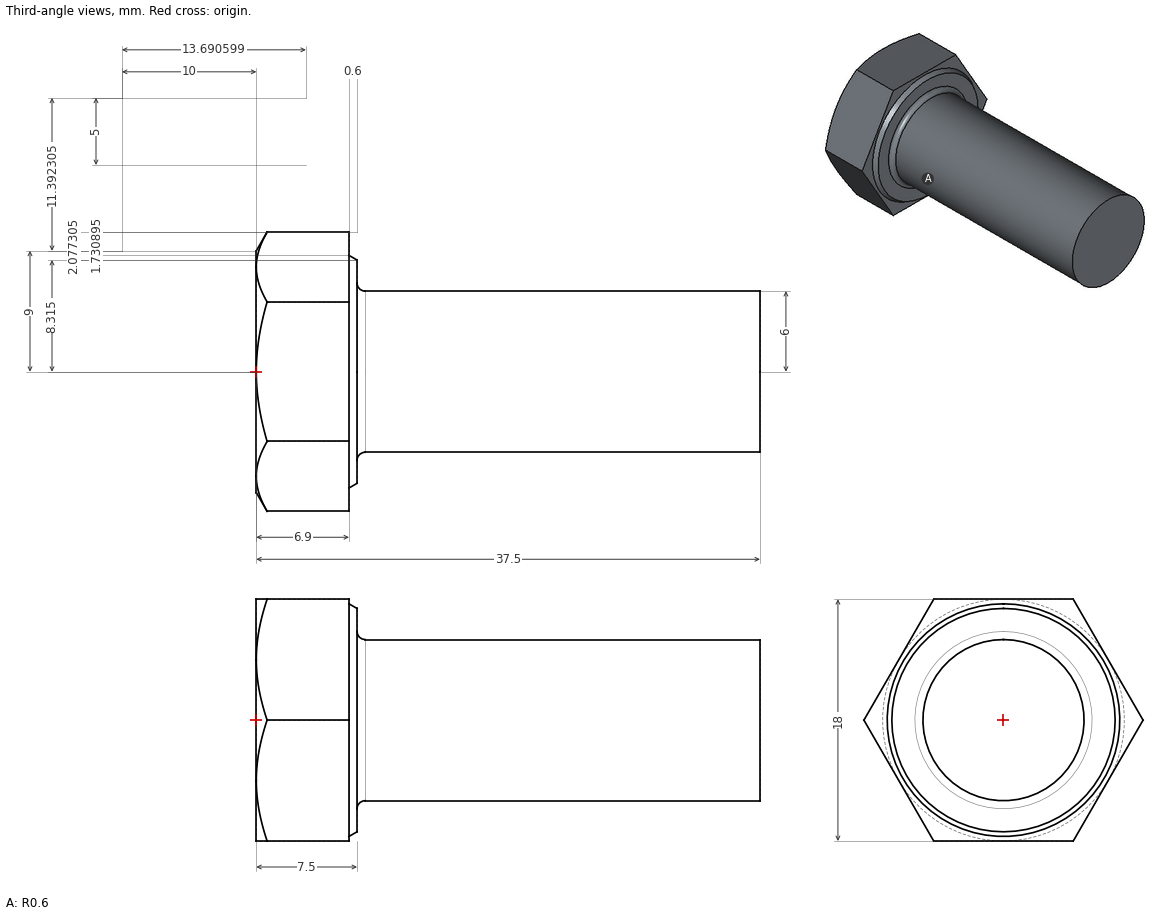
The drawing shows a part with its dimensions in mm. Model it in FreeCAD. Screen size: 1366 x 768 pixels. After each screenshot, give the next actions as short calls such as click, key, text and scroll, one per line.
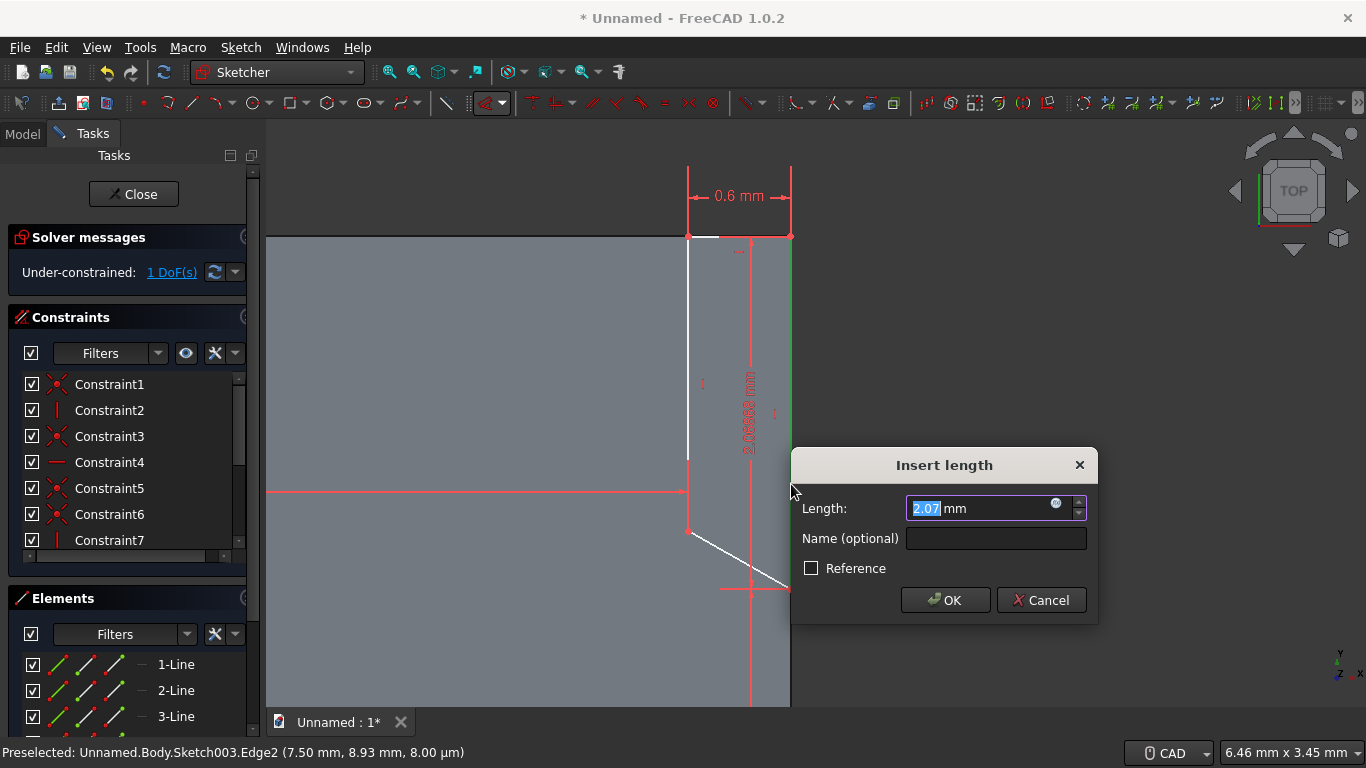
text(2.077305)
key(Return)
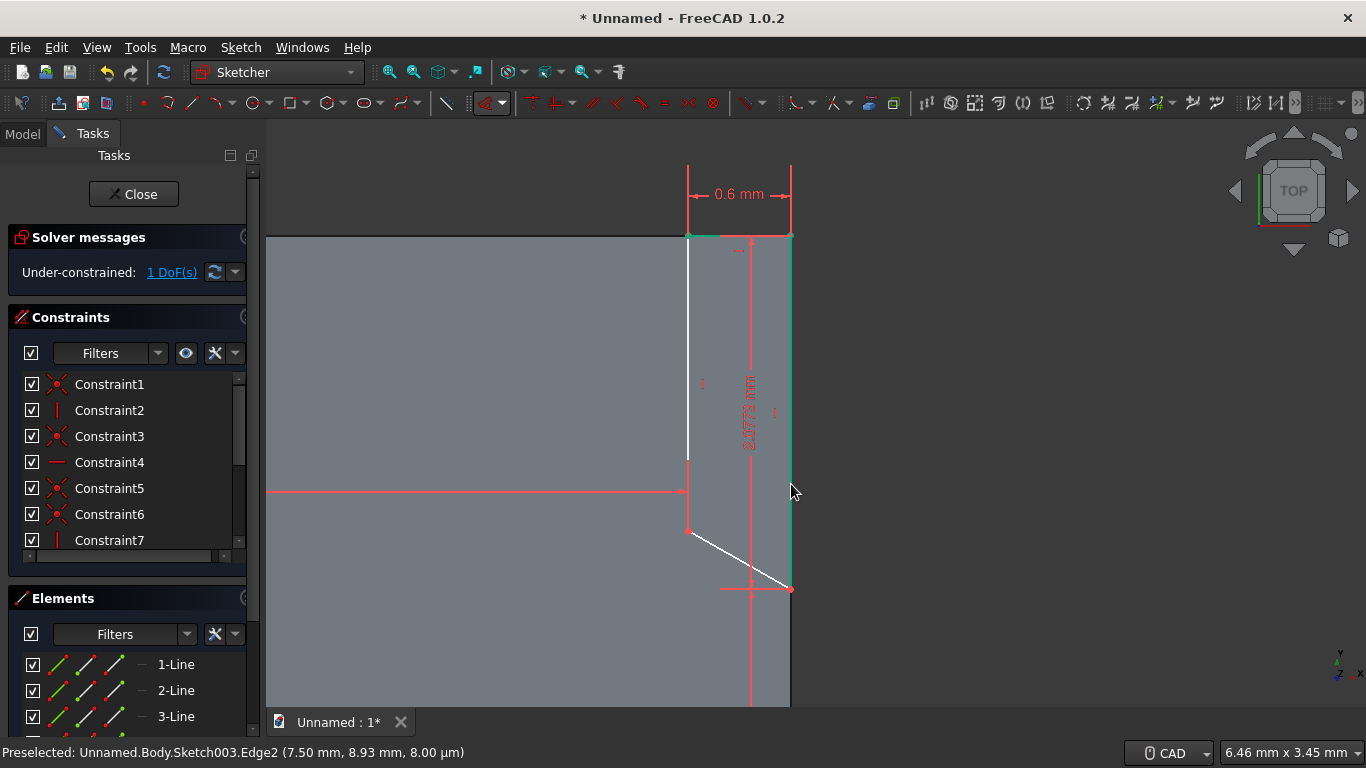
click(688, 324)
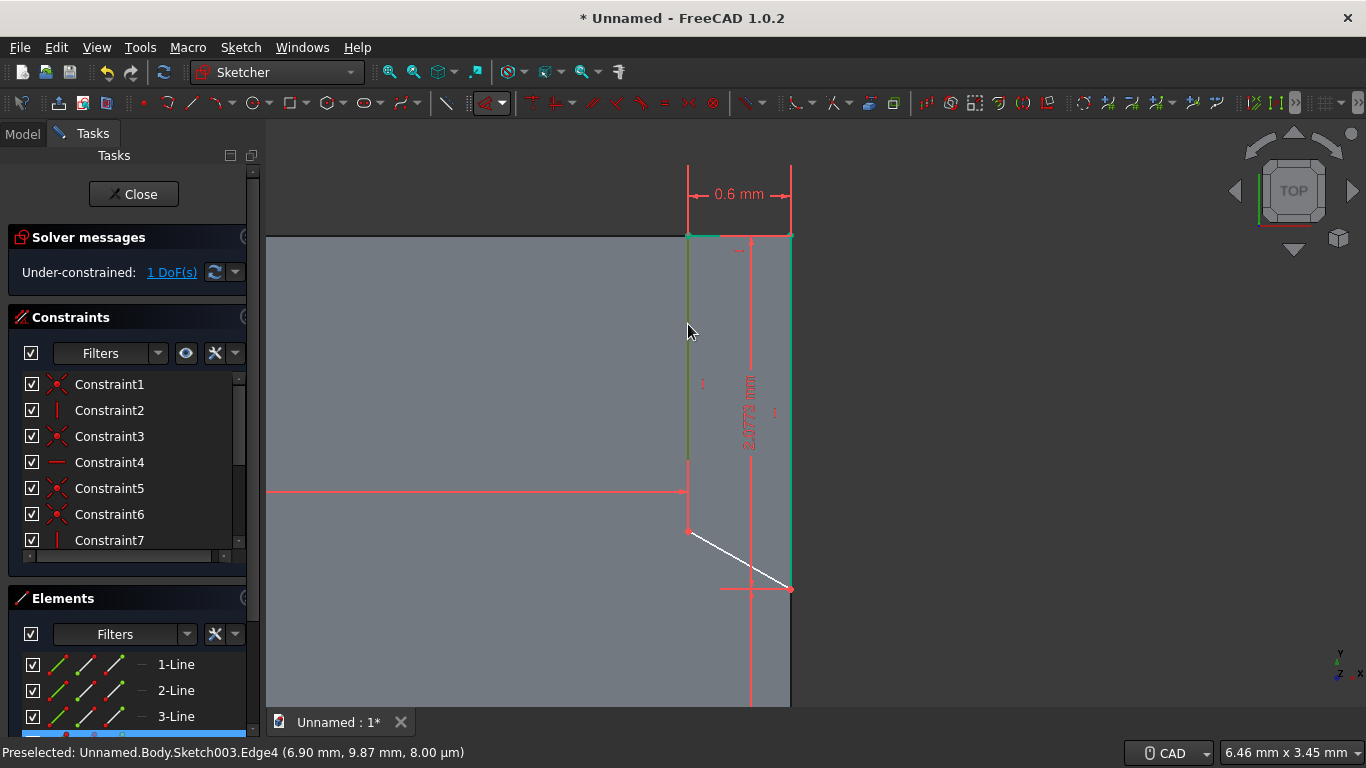
key(i)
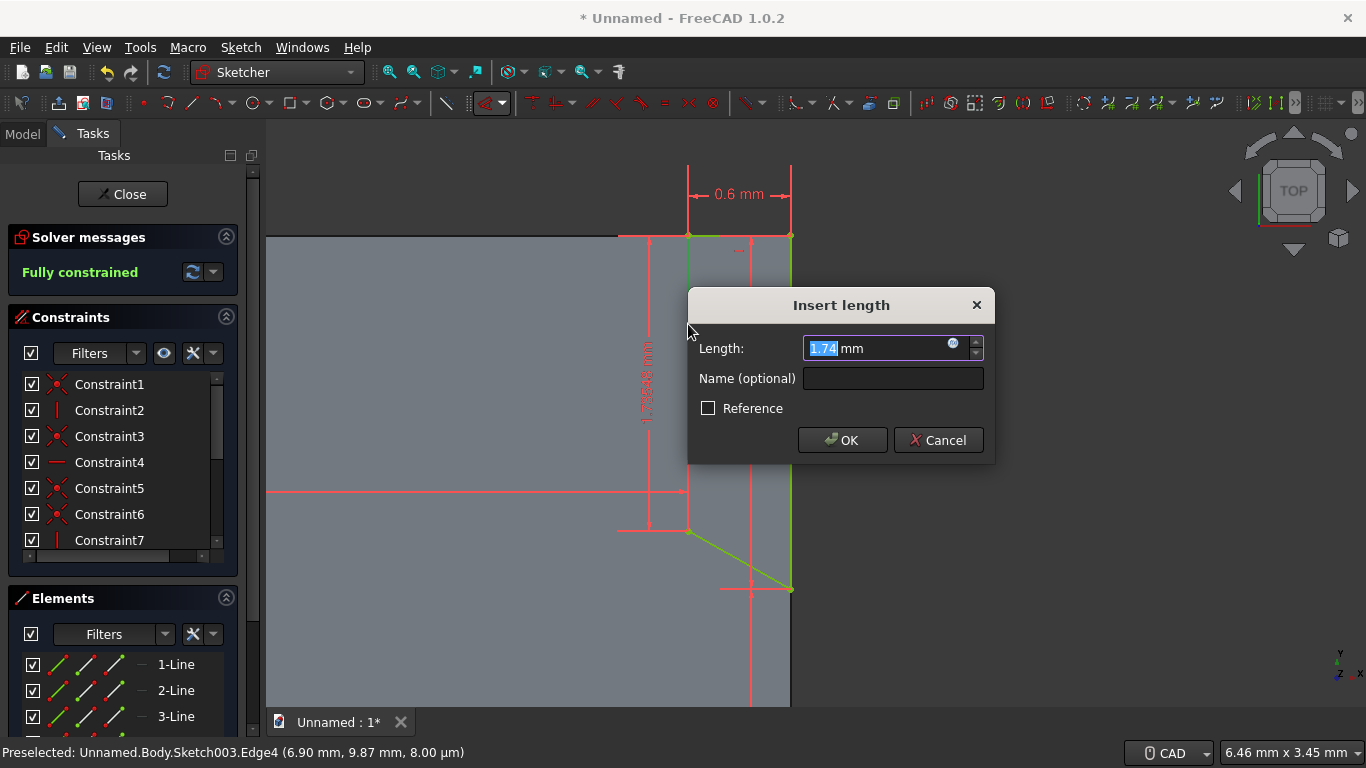
text(1.730895)
key(Return)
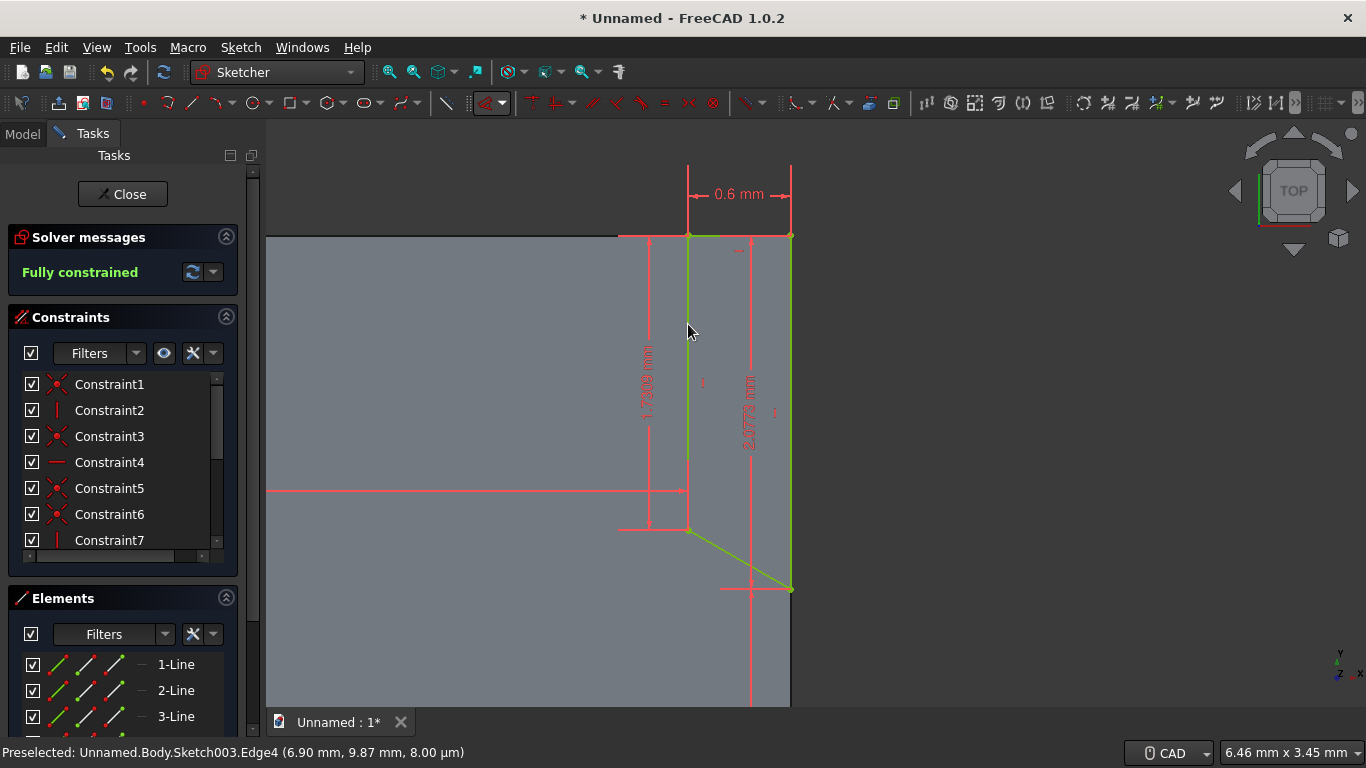
click(123, 194)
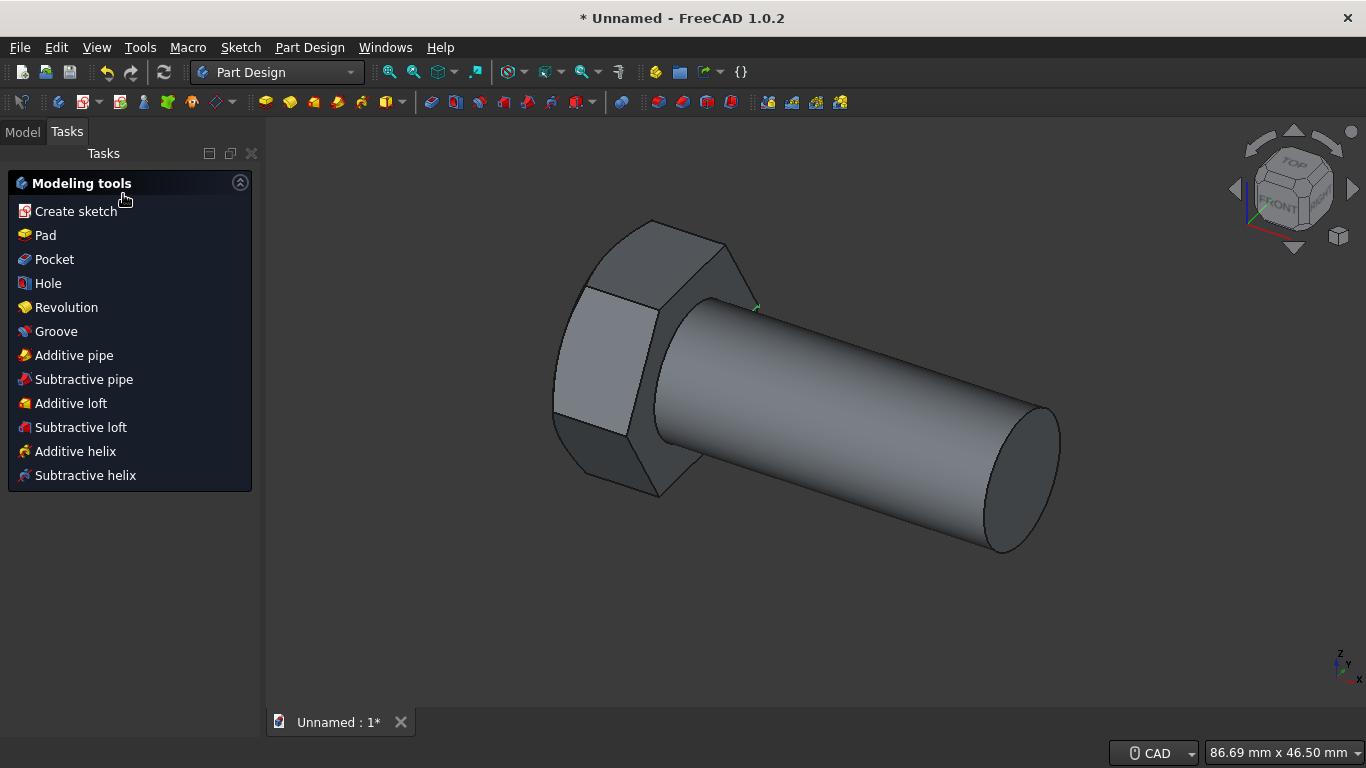
click(480, 102)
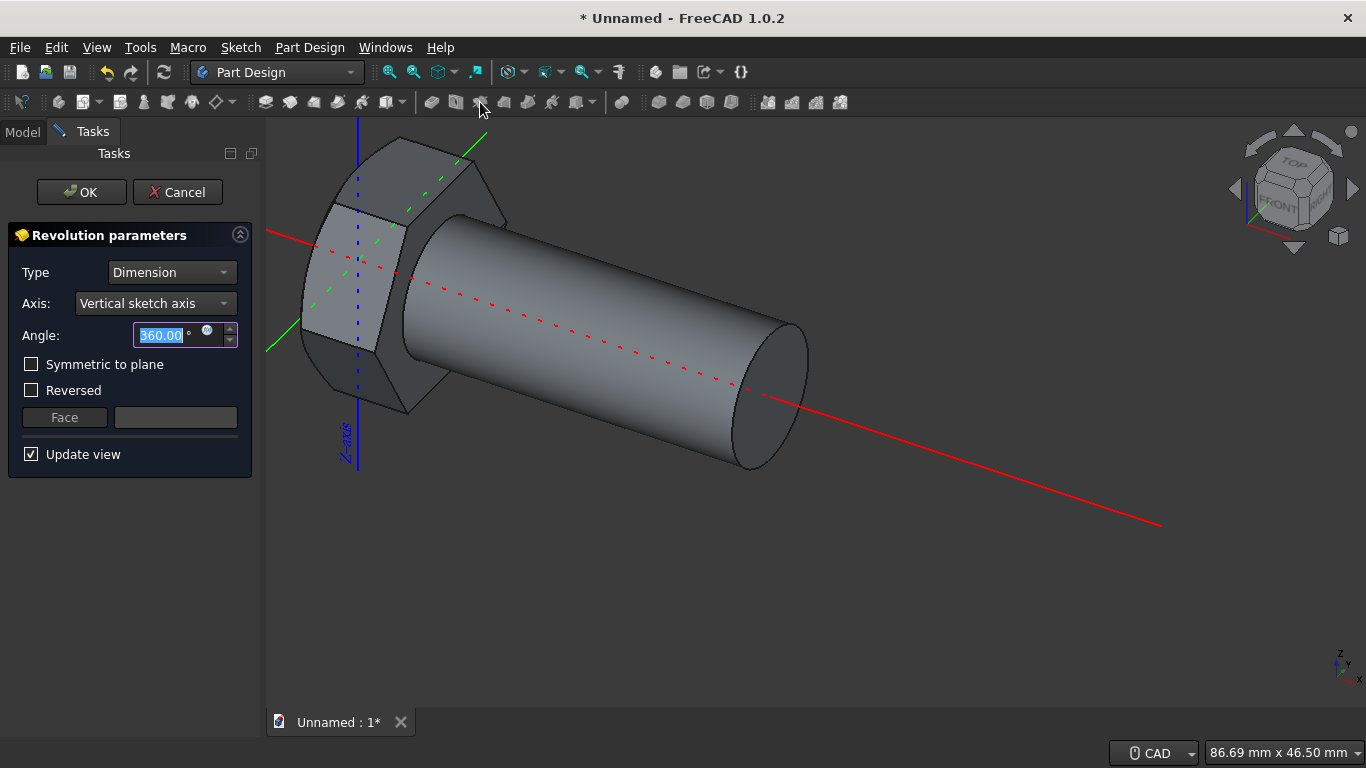
click(156, 304)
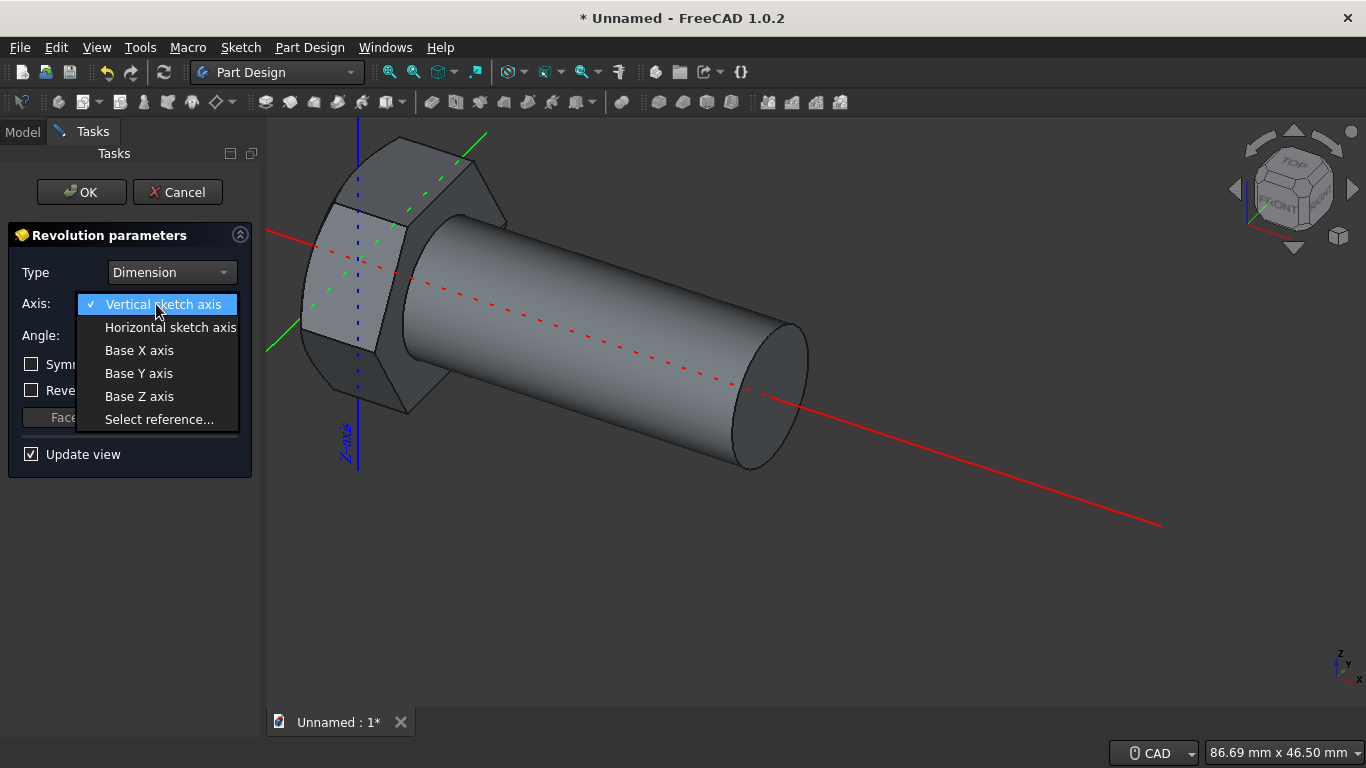
click(156, 328)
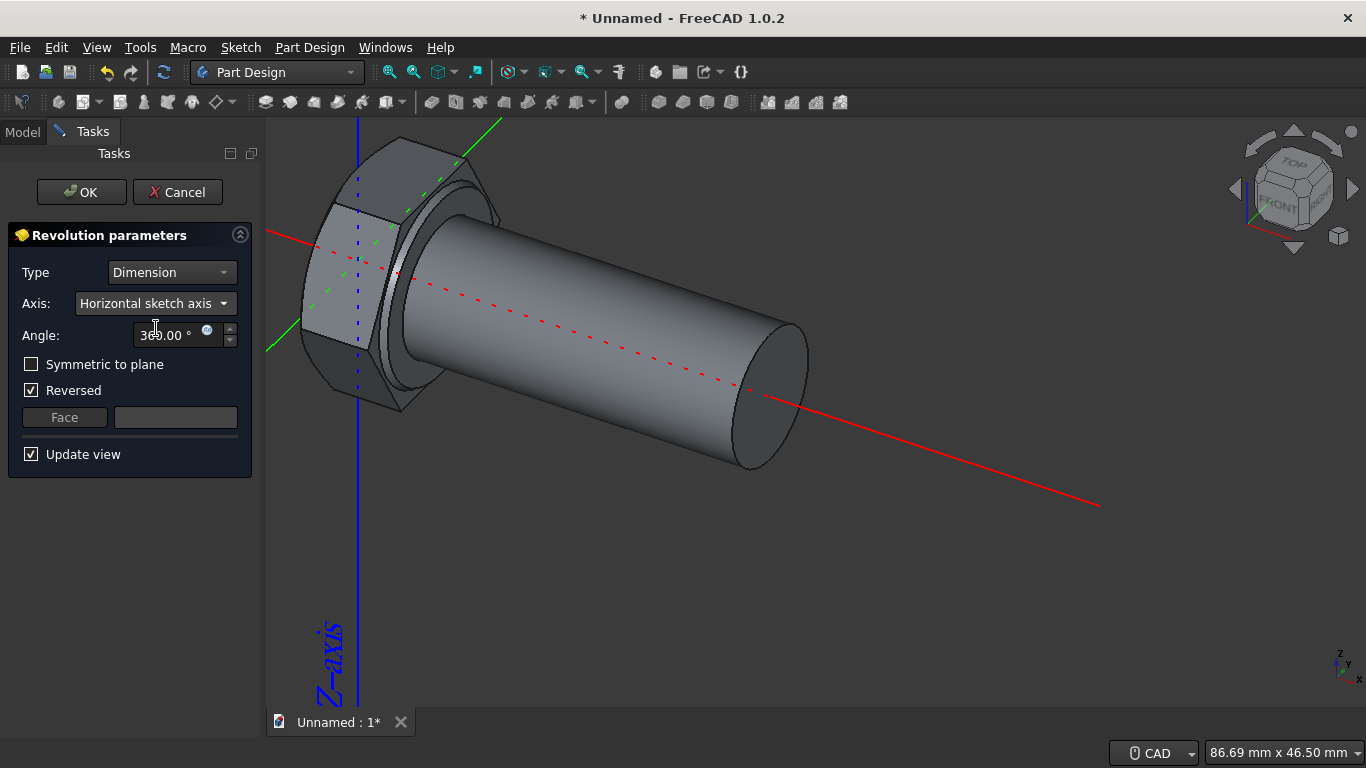
click(82, 192)